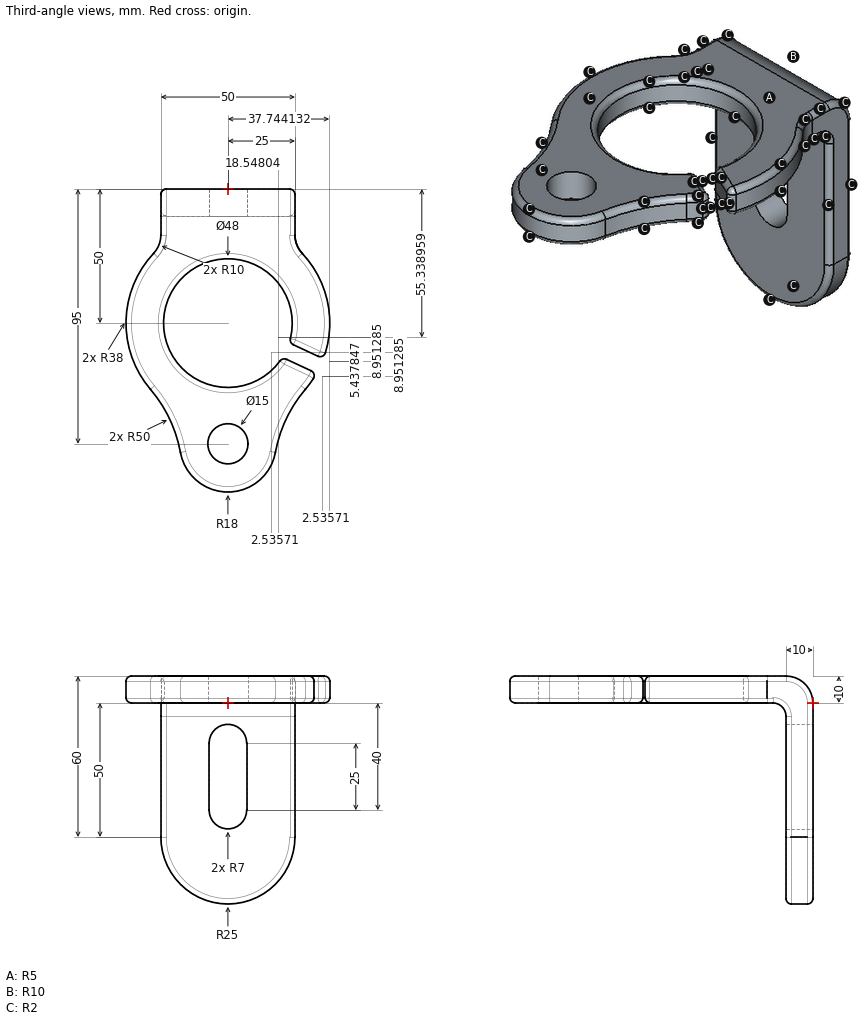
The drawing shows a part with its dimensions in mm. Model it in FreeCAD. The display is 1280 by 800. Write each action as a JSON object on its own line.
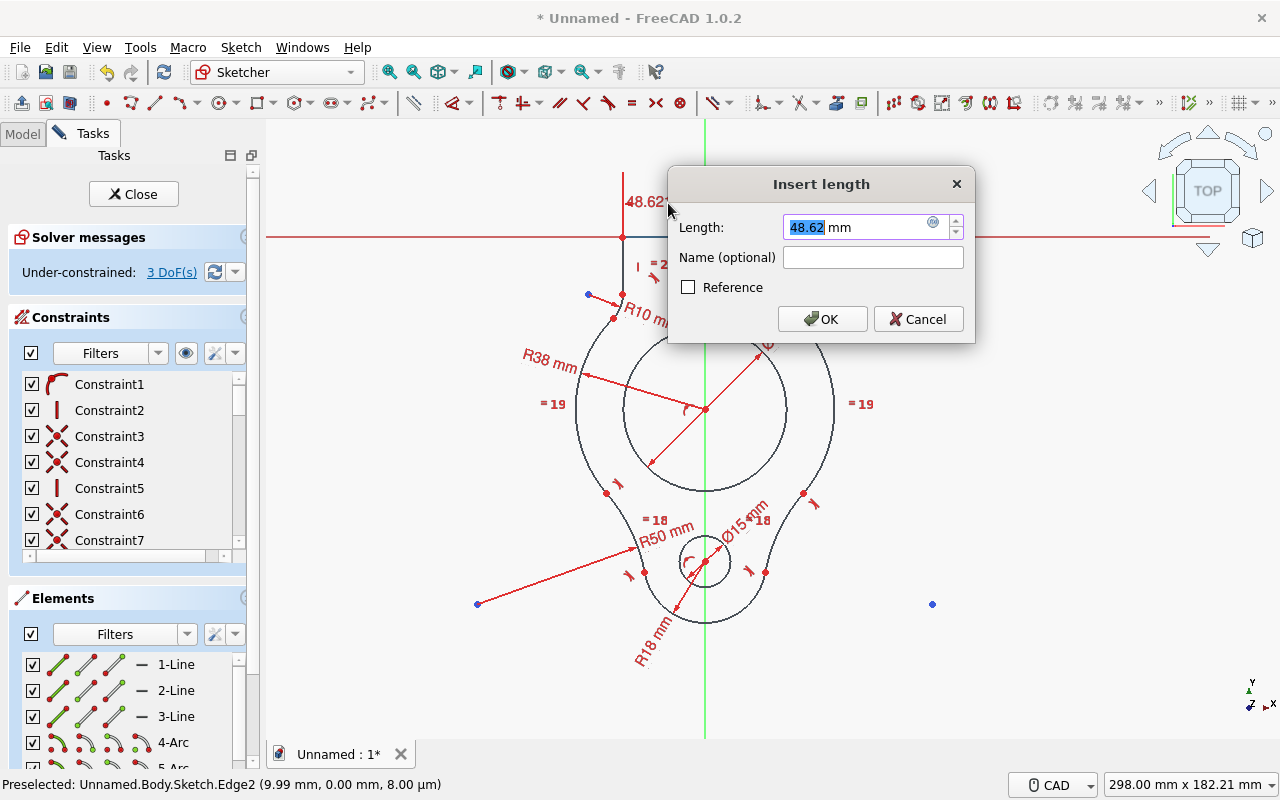
{"action": "type", "text": "50"}
{"action": "key", "text": "Return"}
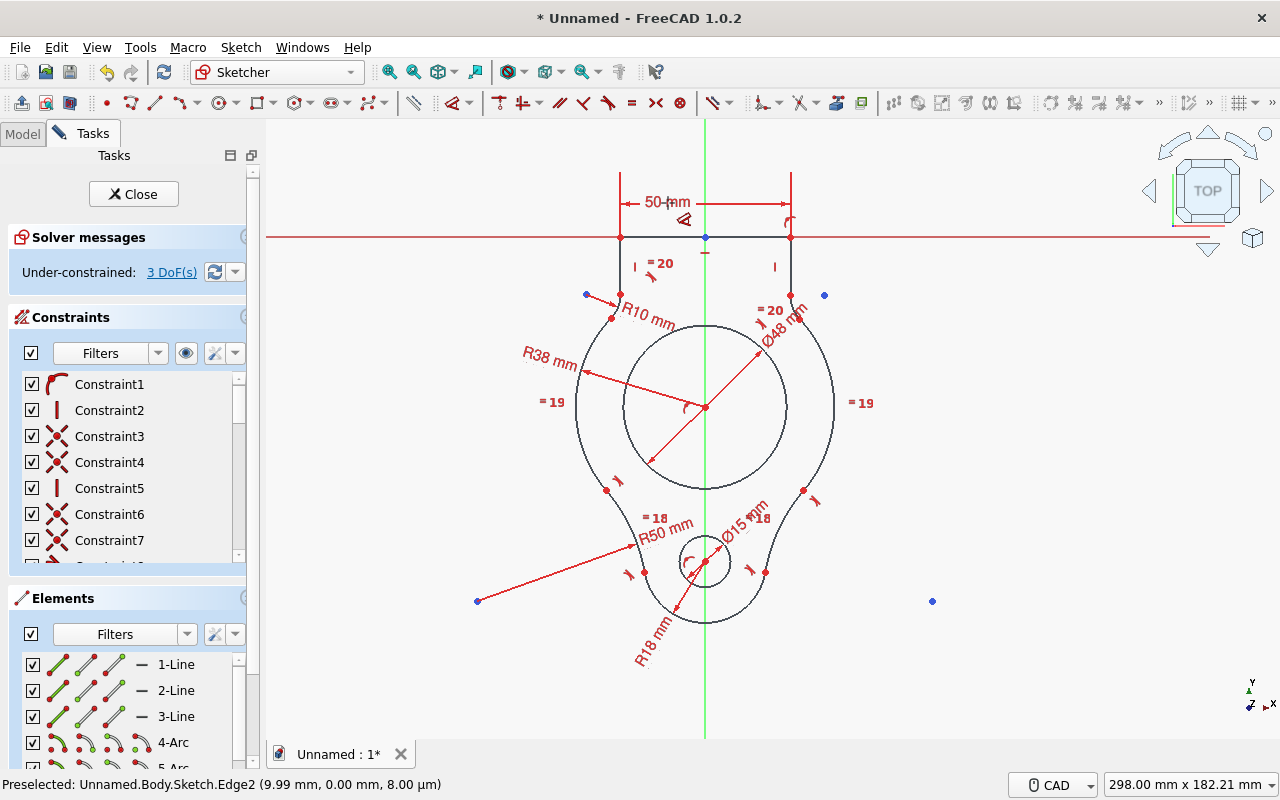
{"action": "left_click", "coordinate": [705, 562]}
{"action": "left_click", "coordinate": [739, 399]}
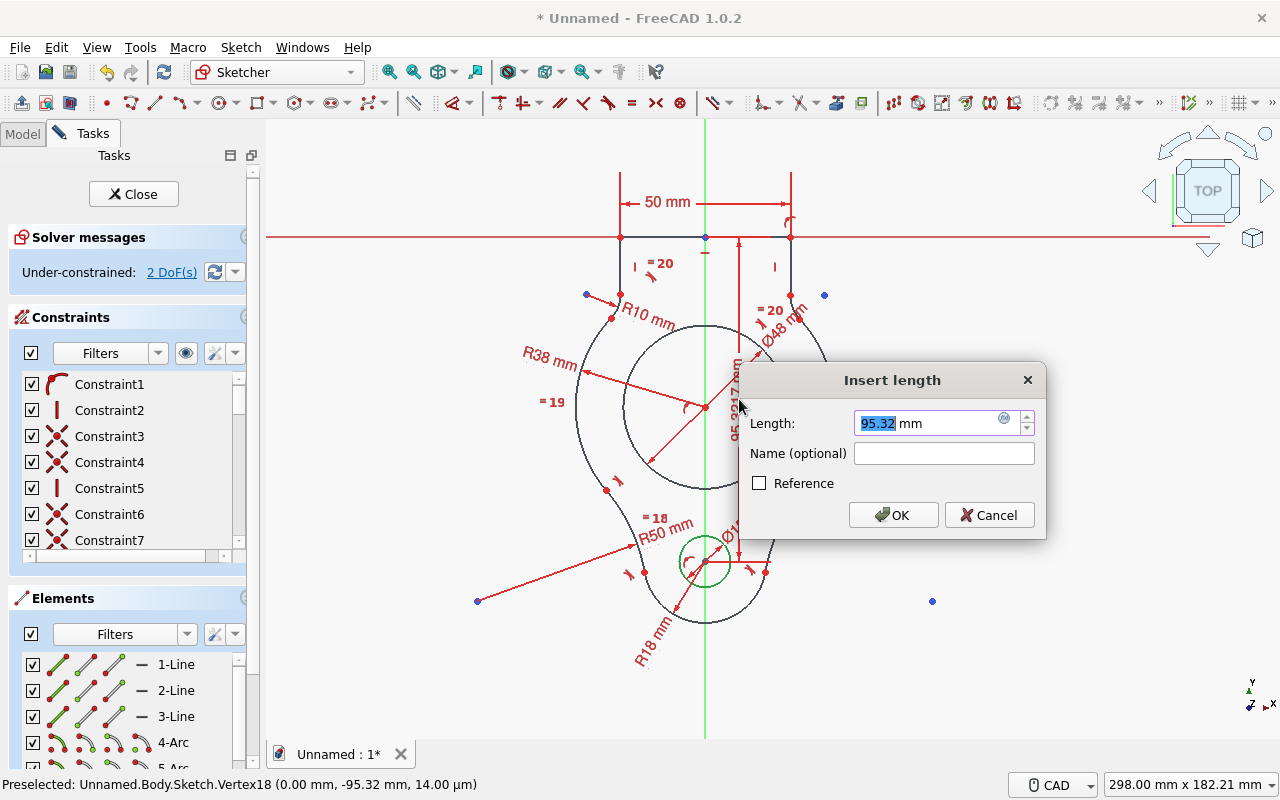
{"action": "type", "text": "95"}
{"action": "key", "text": "Return"}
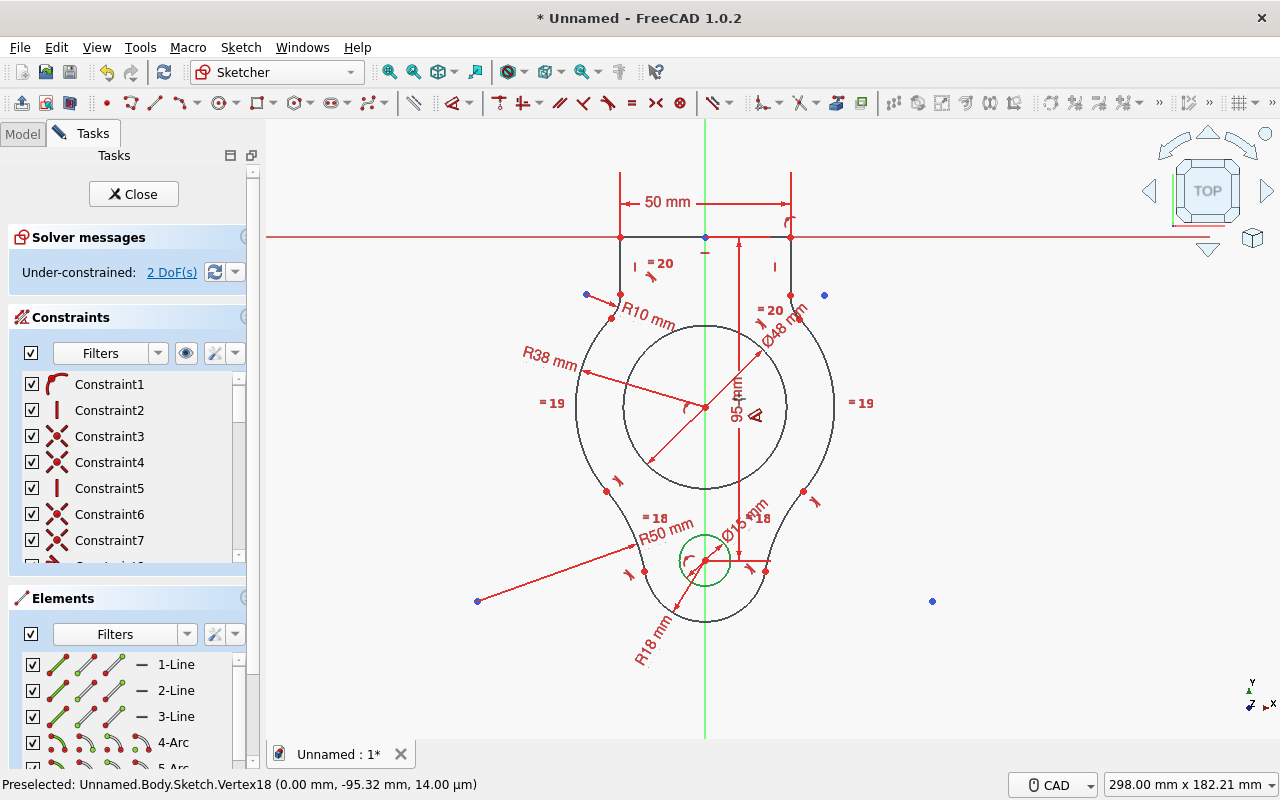
{"action": "left_click", "coordinate": [705, 407]}
{"action": "left_click", "coordinate": [739, 283]}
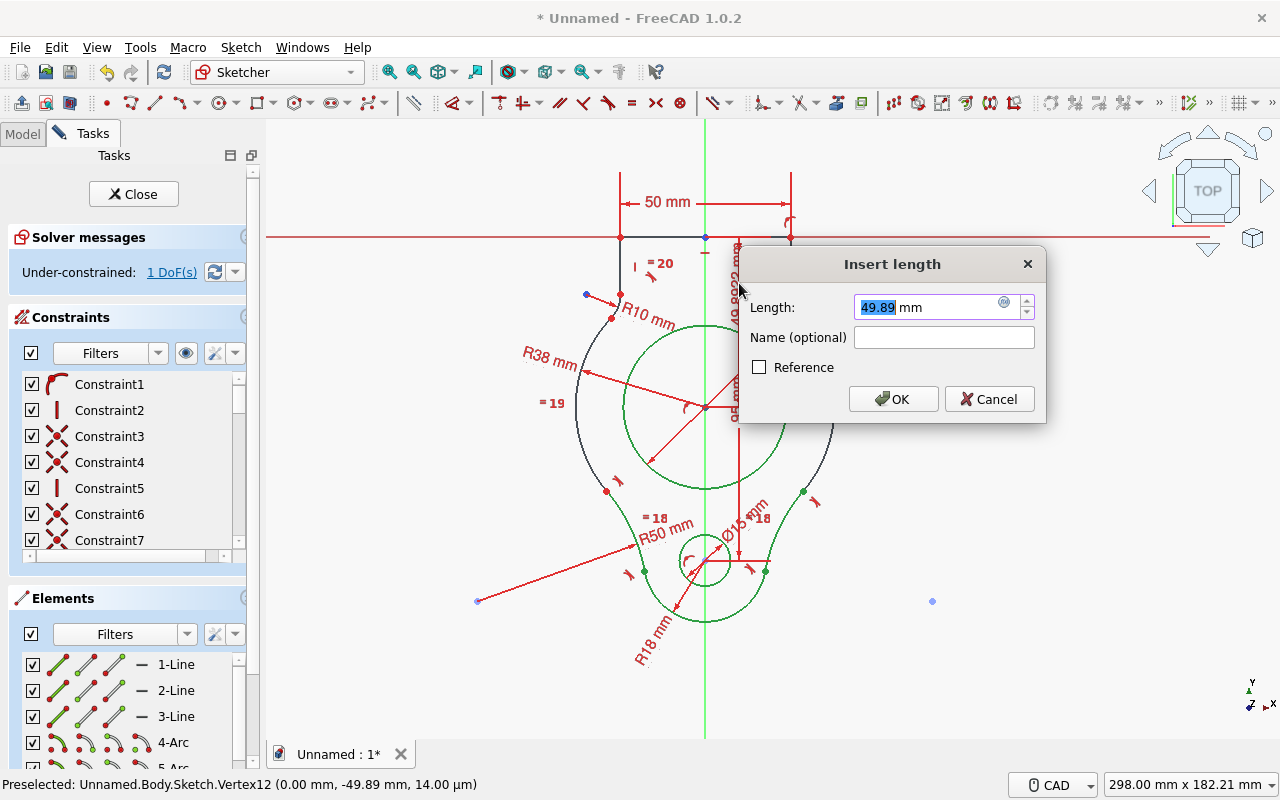
{"action": "type", "text": "50"}
{"action": "key", "text": "Return"}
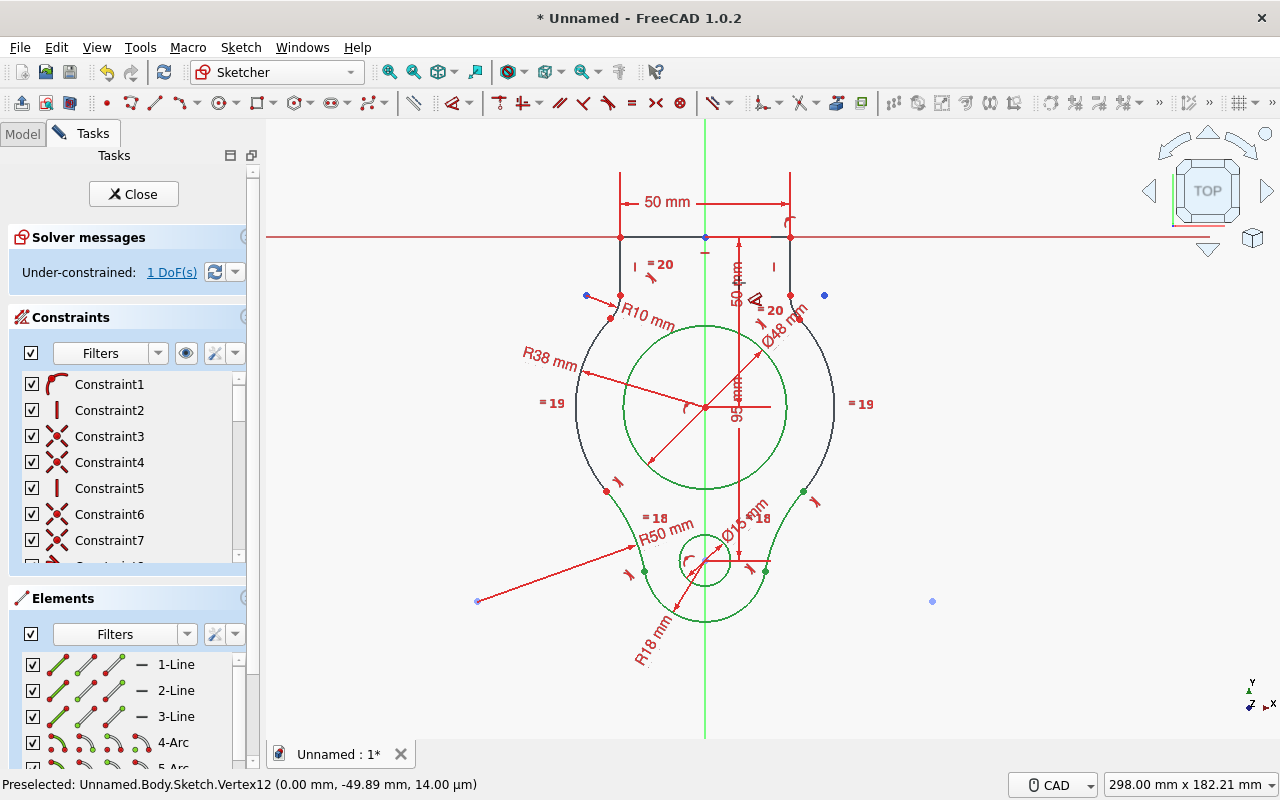
{"action": "left_click", "coordinate": [790, 296]}
{"action": "left_click", "coordinate": [748, 203]}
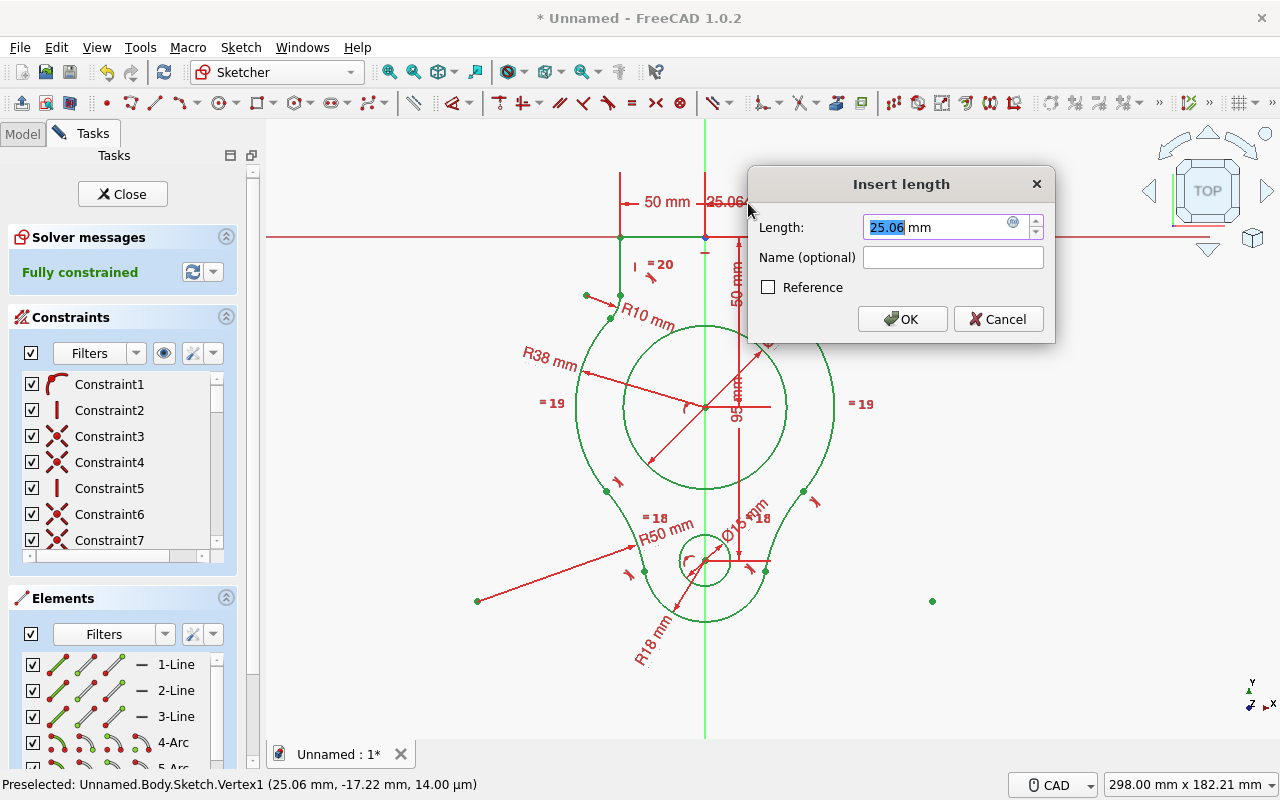
{"action": "type", "text": "25"}
{"action": "key", "text": "Return"}
{"action": "key", "text": "Escape"}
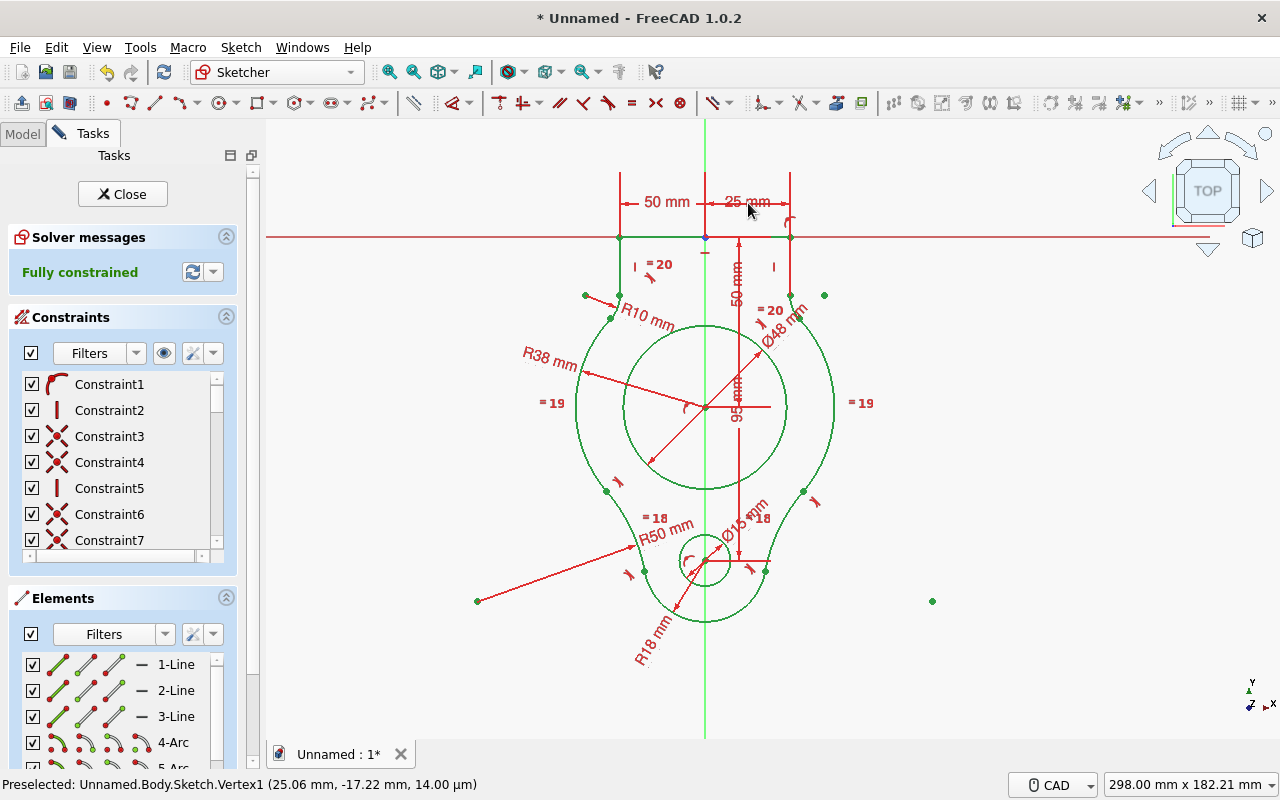
{"action": "left_click", "coordinate": [123, 194]}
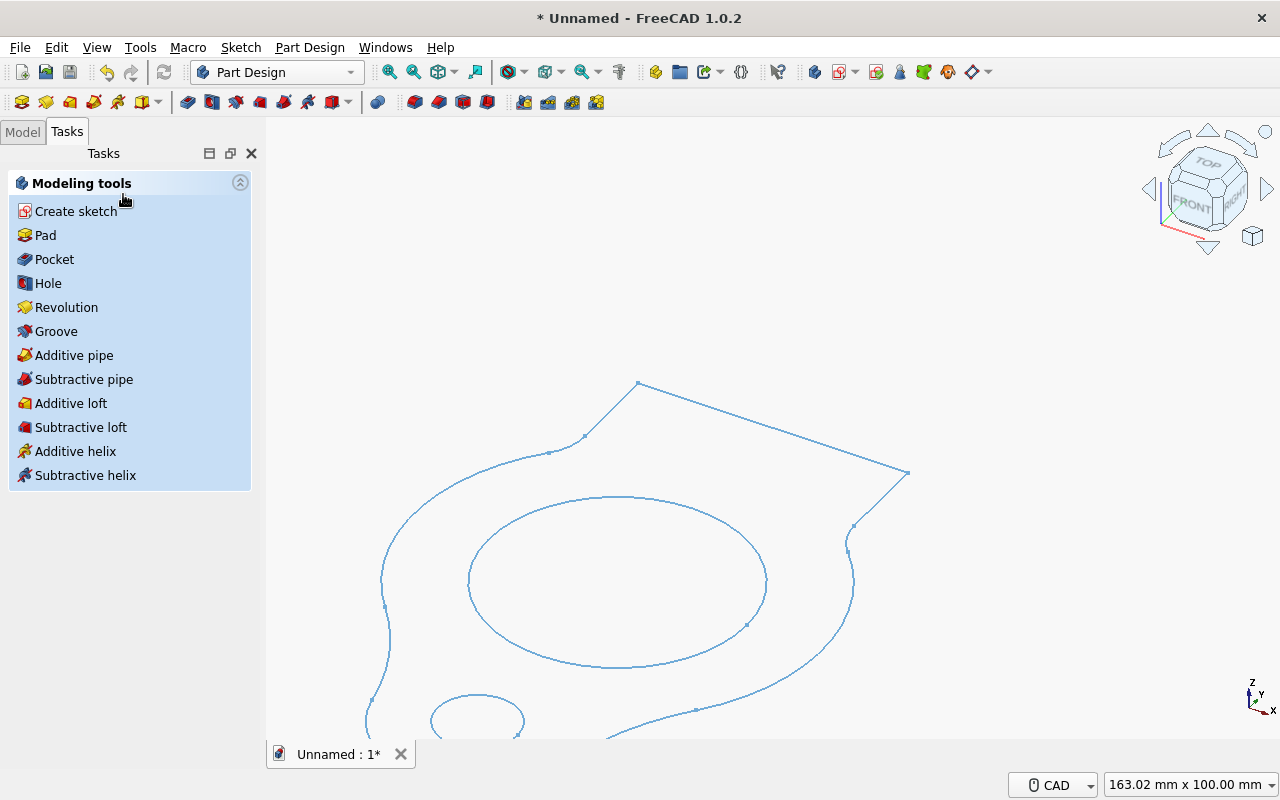
{"action": "left_click", "coordinate": [22, 102]}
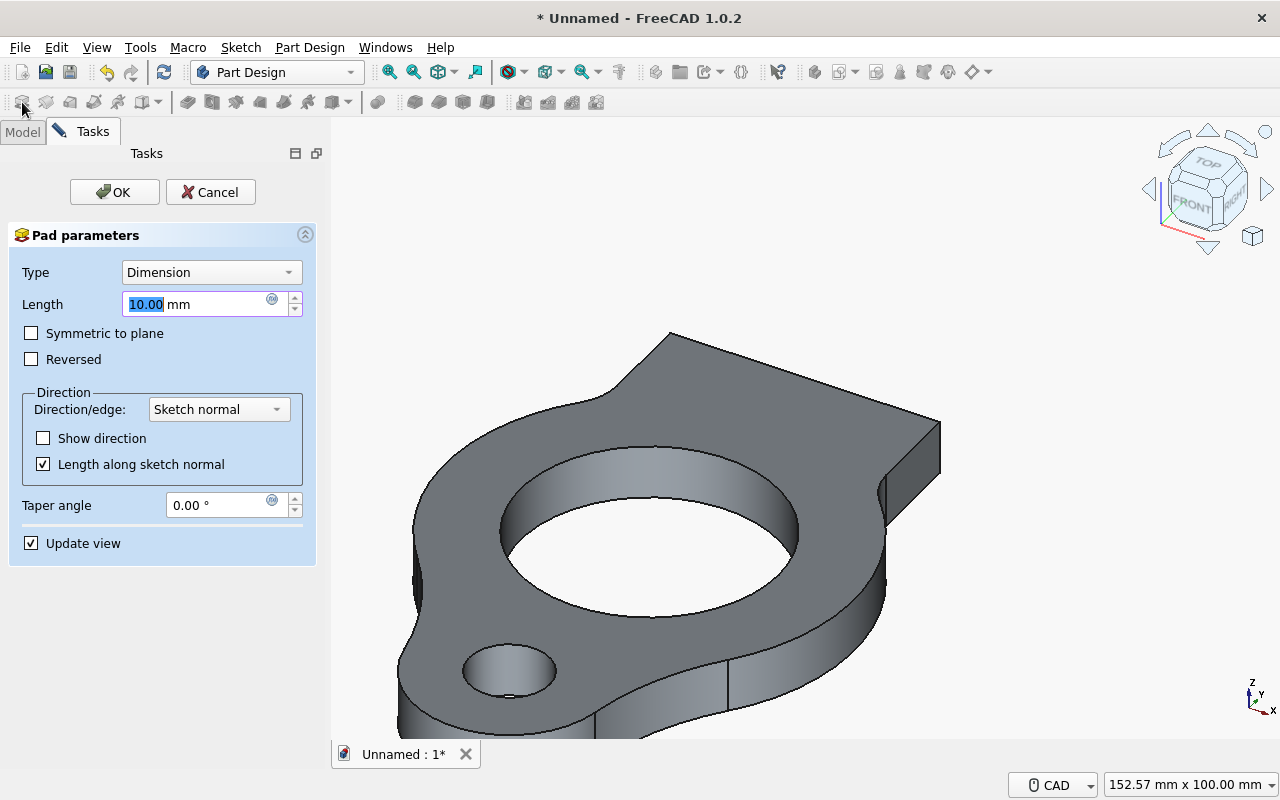
{"action": "type", "text": "10"}
{"action": "key", "text": "Tab"}